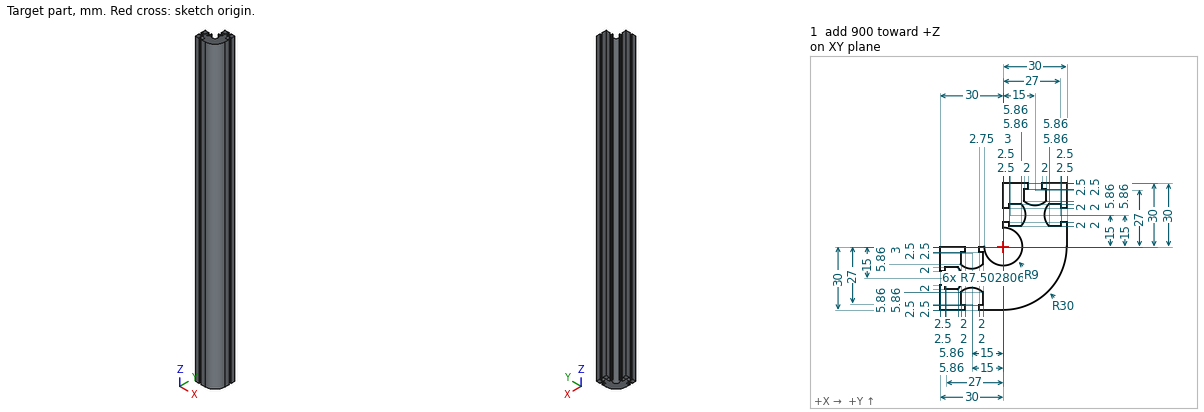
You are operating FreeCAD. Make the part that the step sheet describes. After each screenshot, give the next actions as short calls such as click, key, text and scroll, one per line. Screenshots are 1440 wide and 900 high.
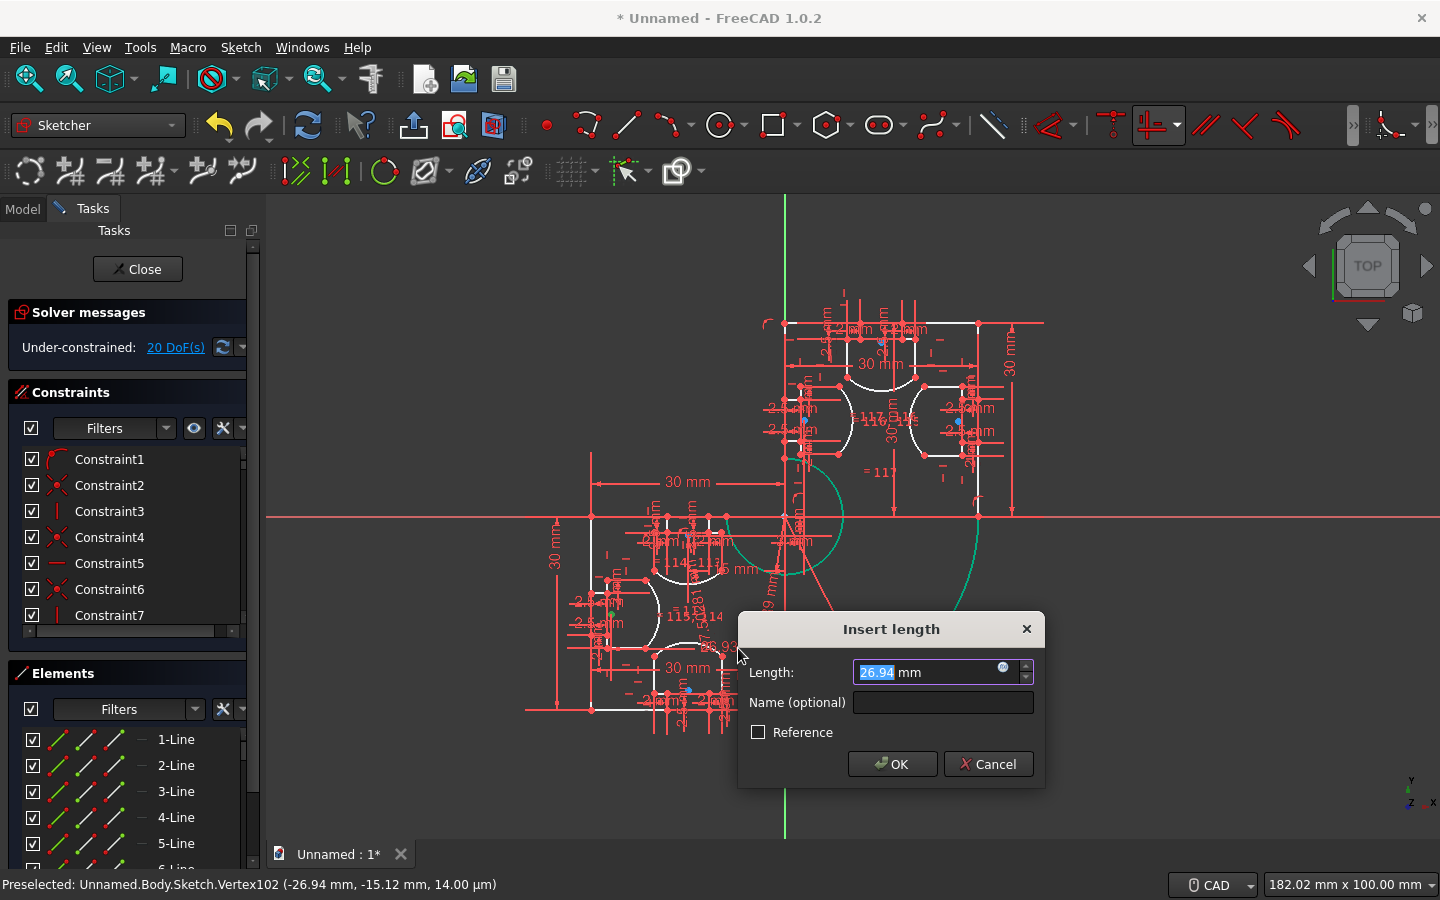
text(27)
key(Return)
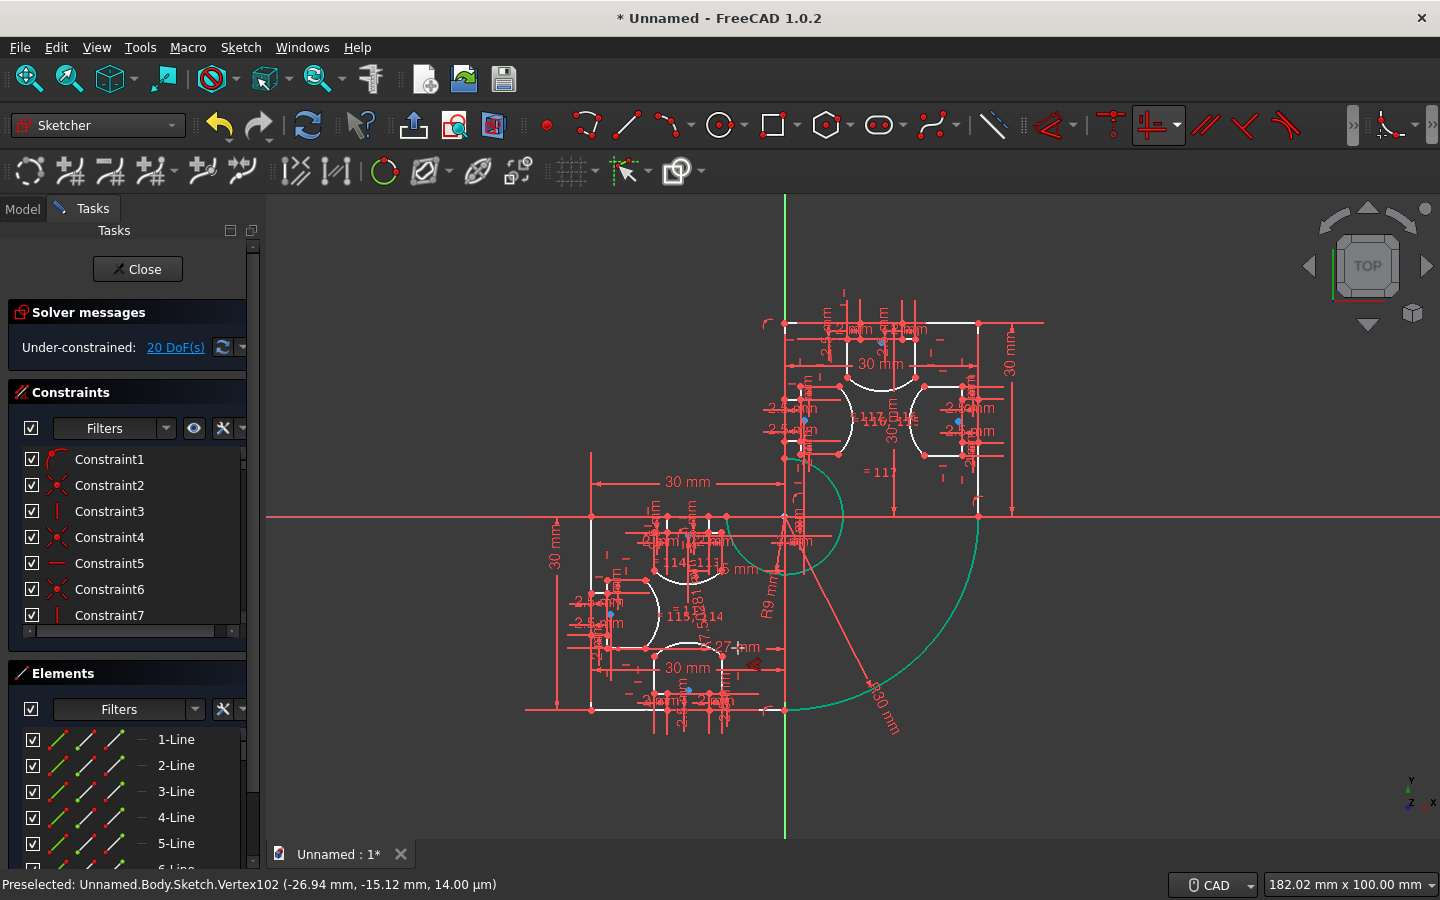
click(611, 614)
click(843, 565)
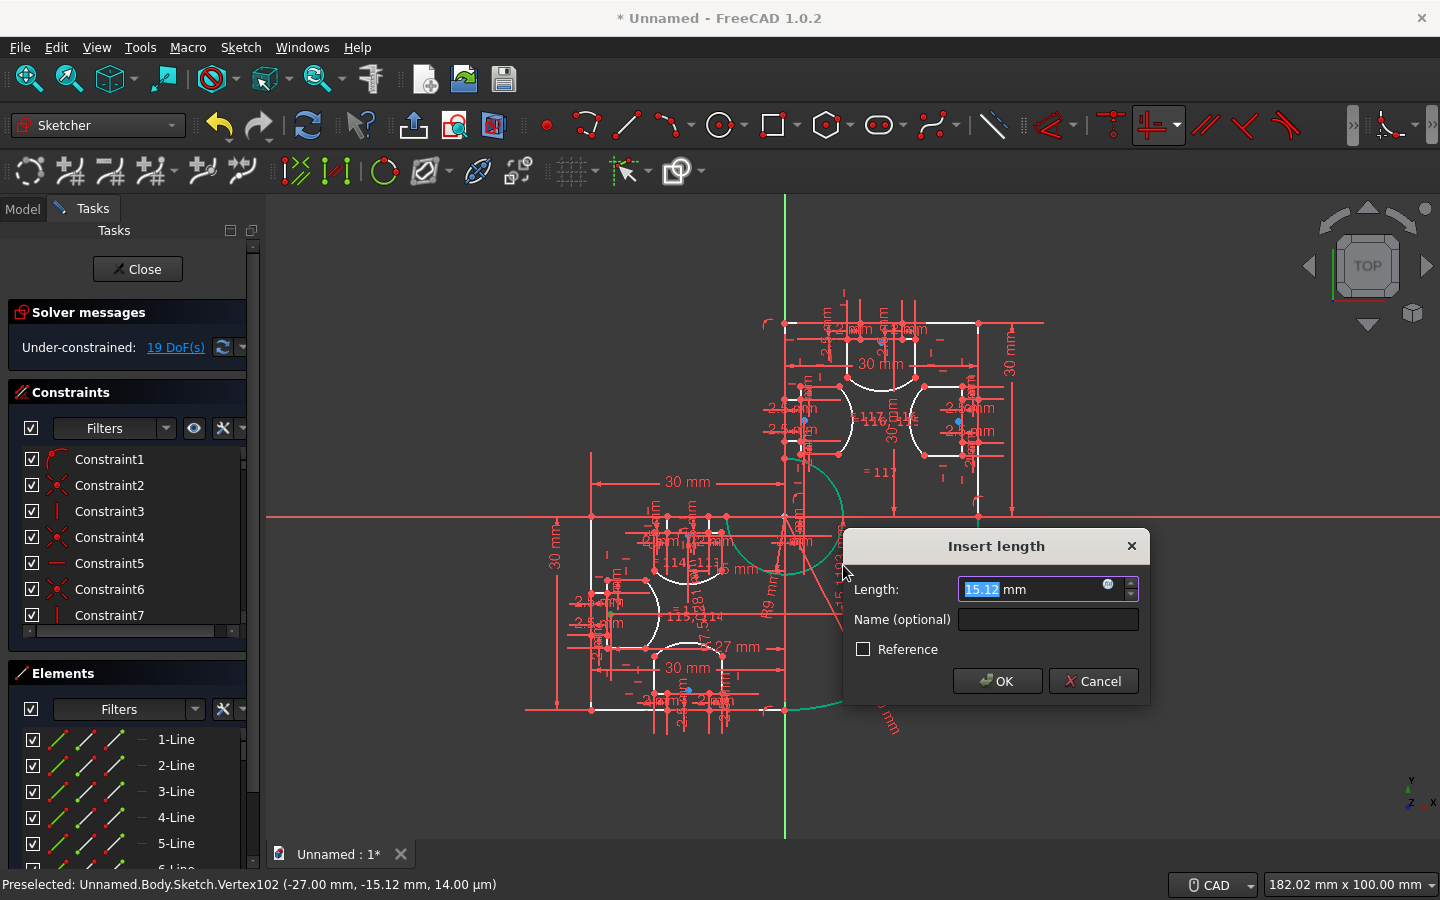
text(15)
key(Return)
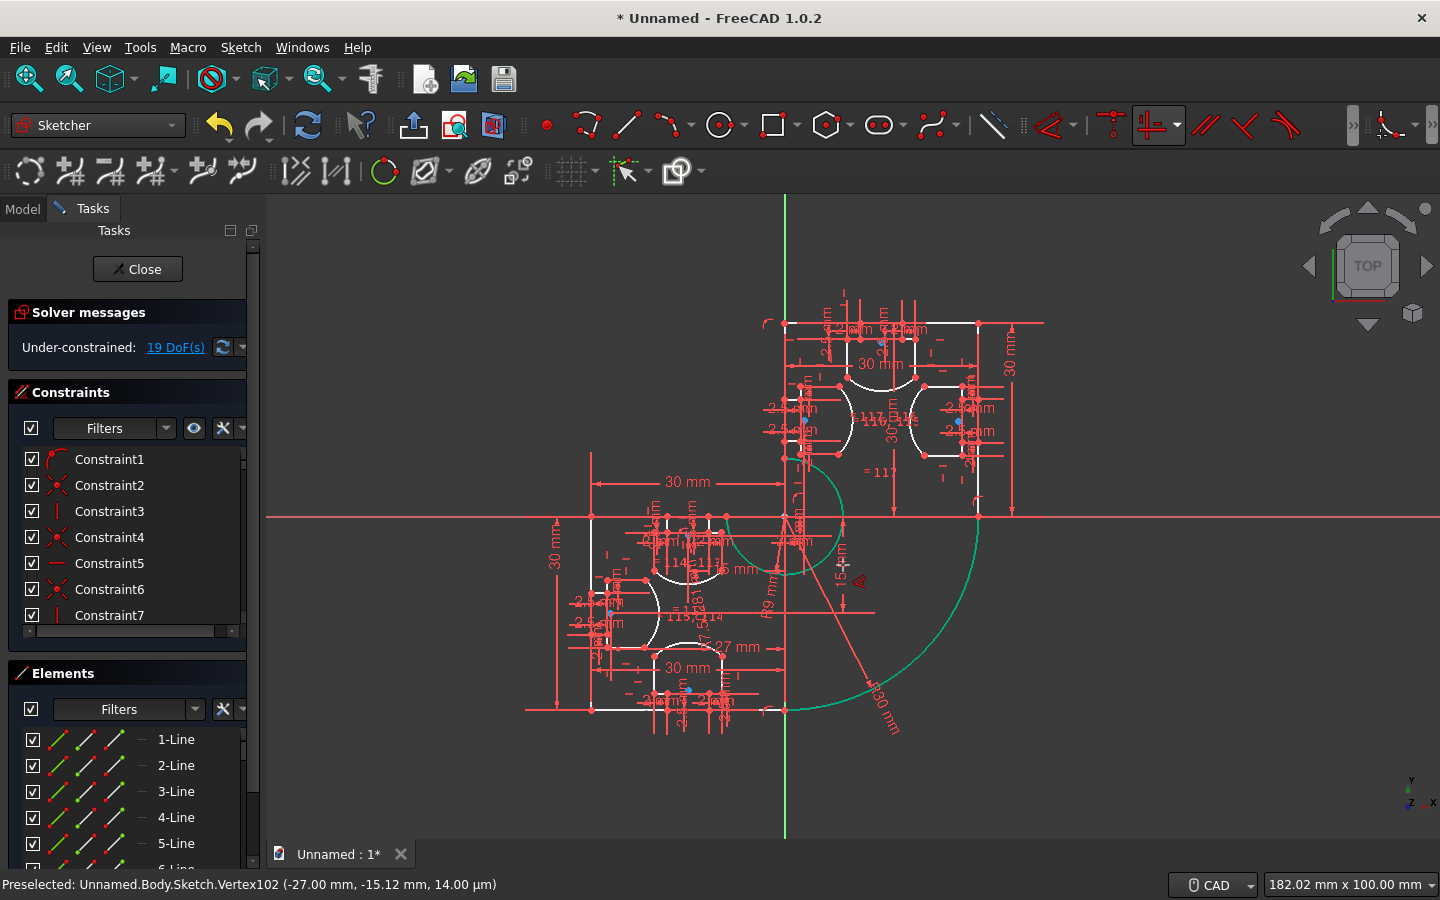
click(688, 691)
click(737, 725)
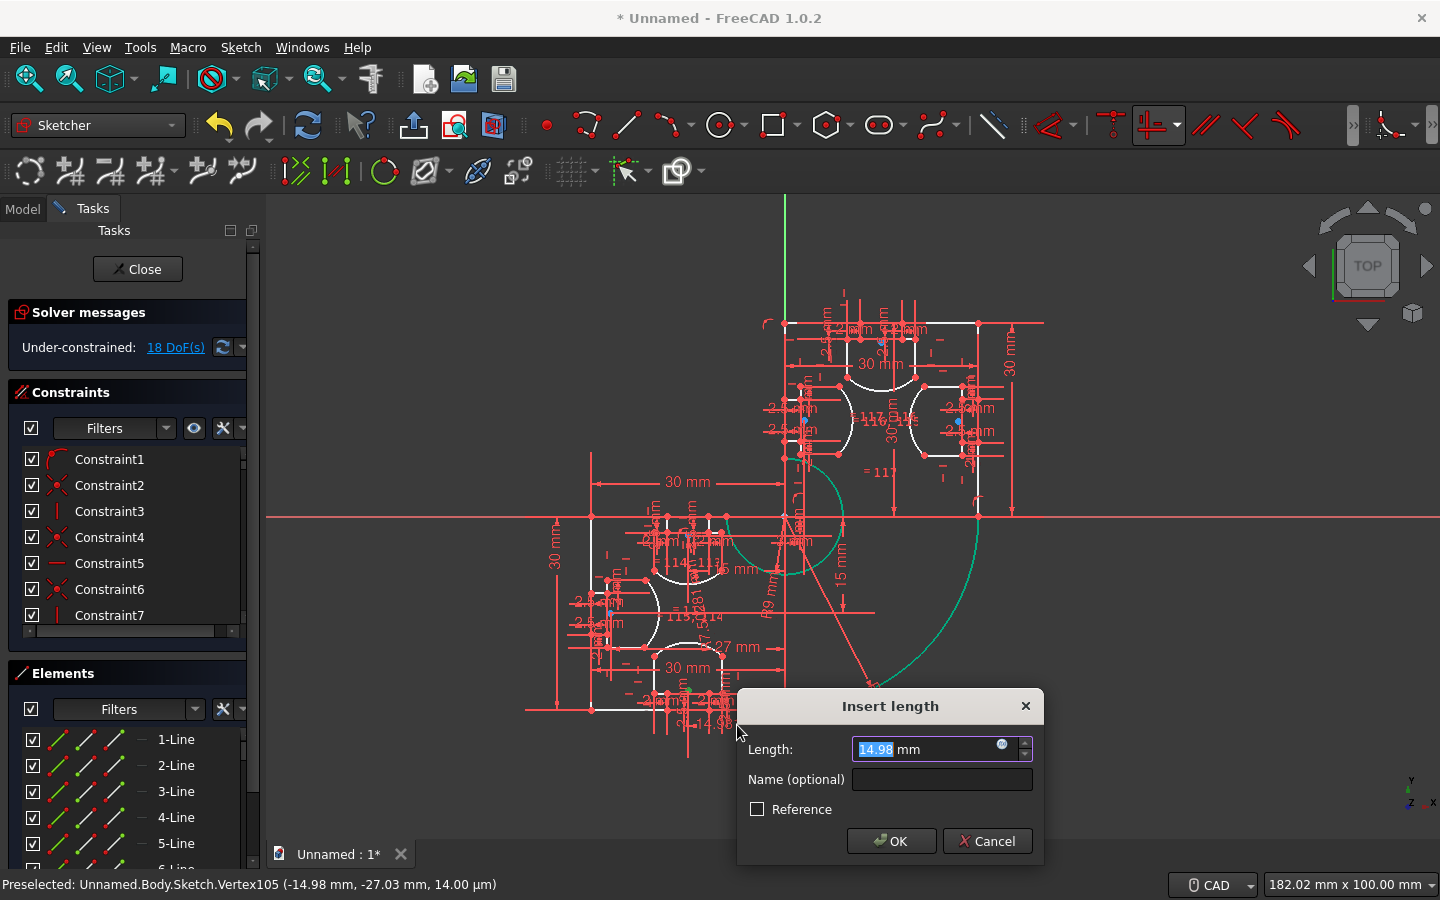
text(15)
key(Return)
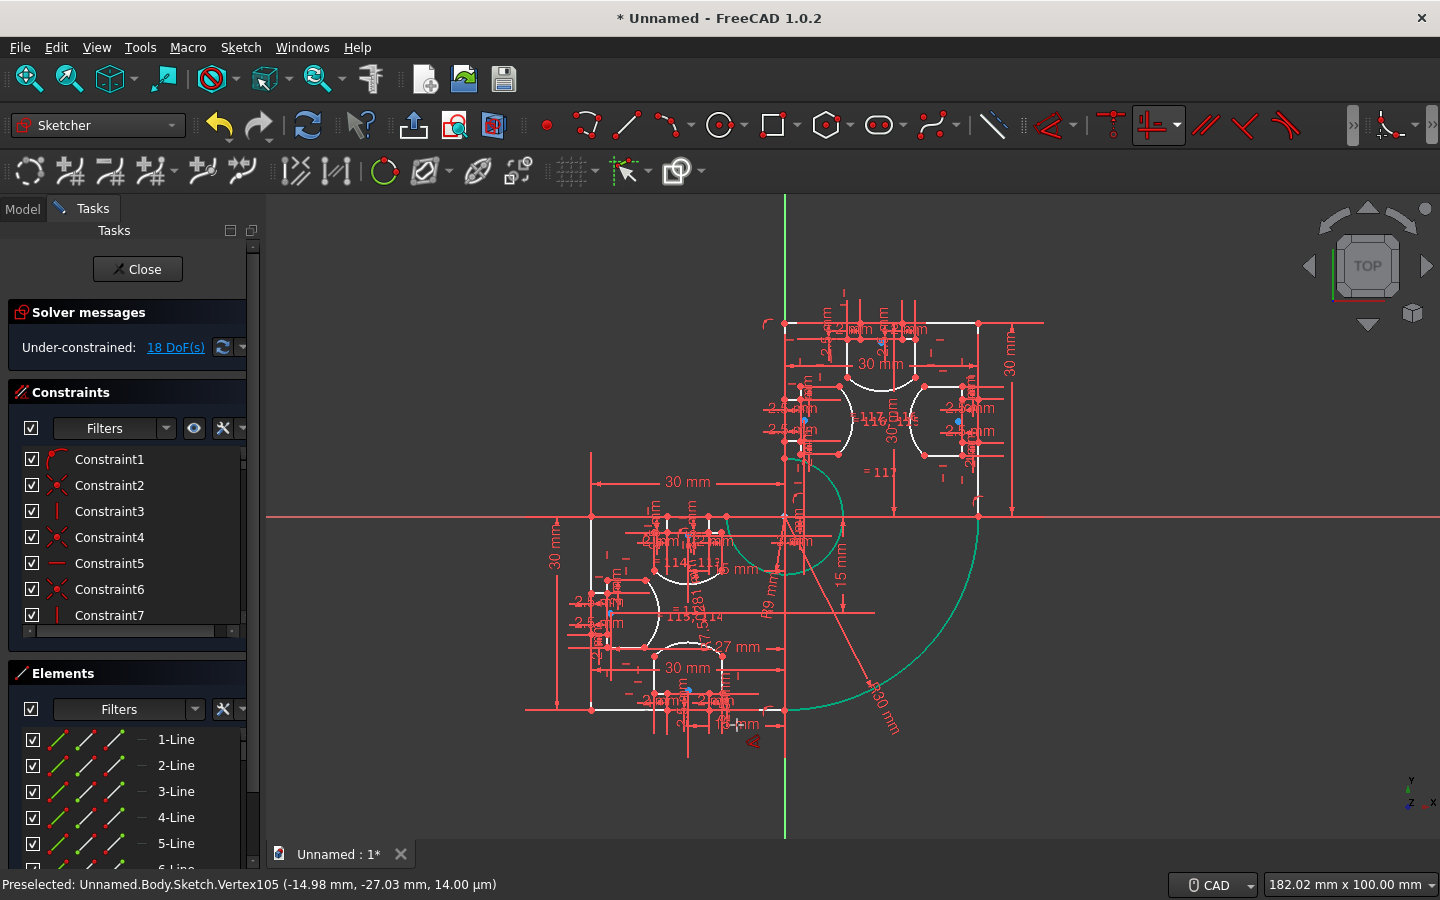
click(688, 691)
click(819, 644)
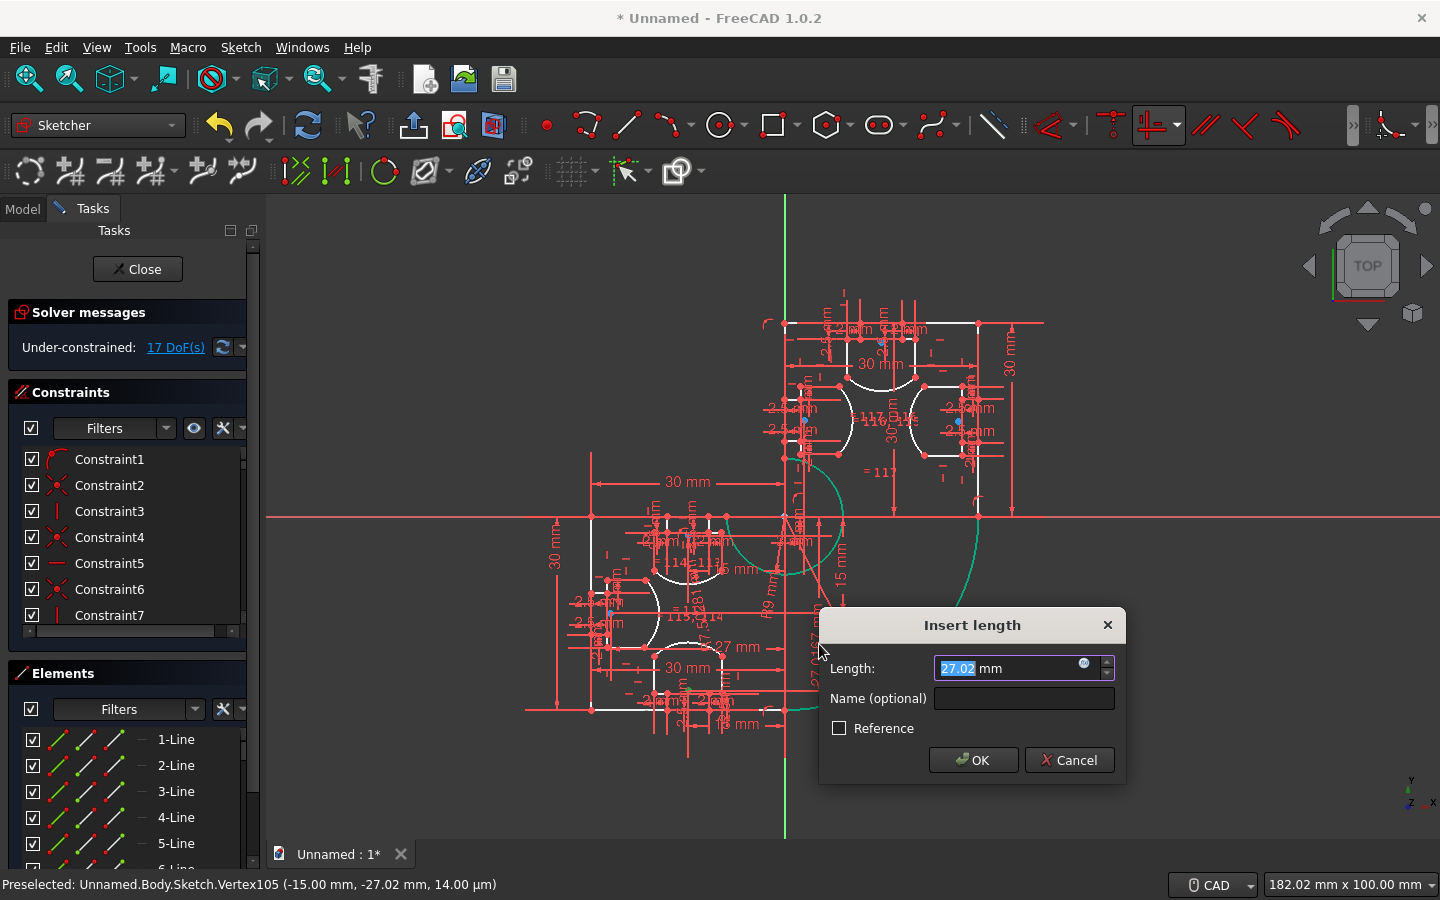
text(27)
key(Return)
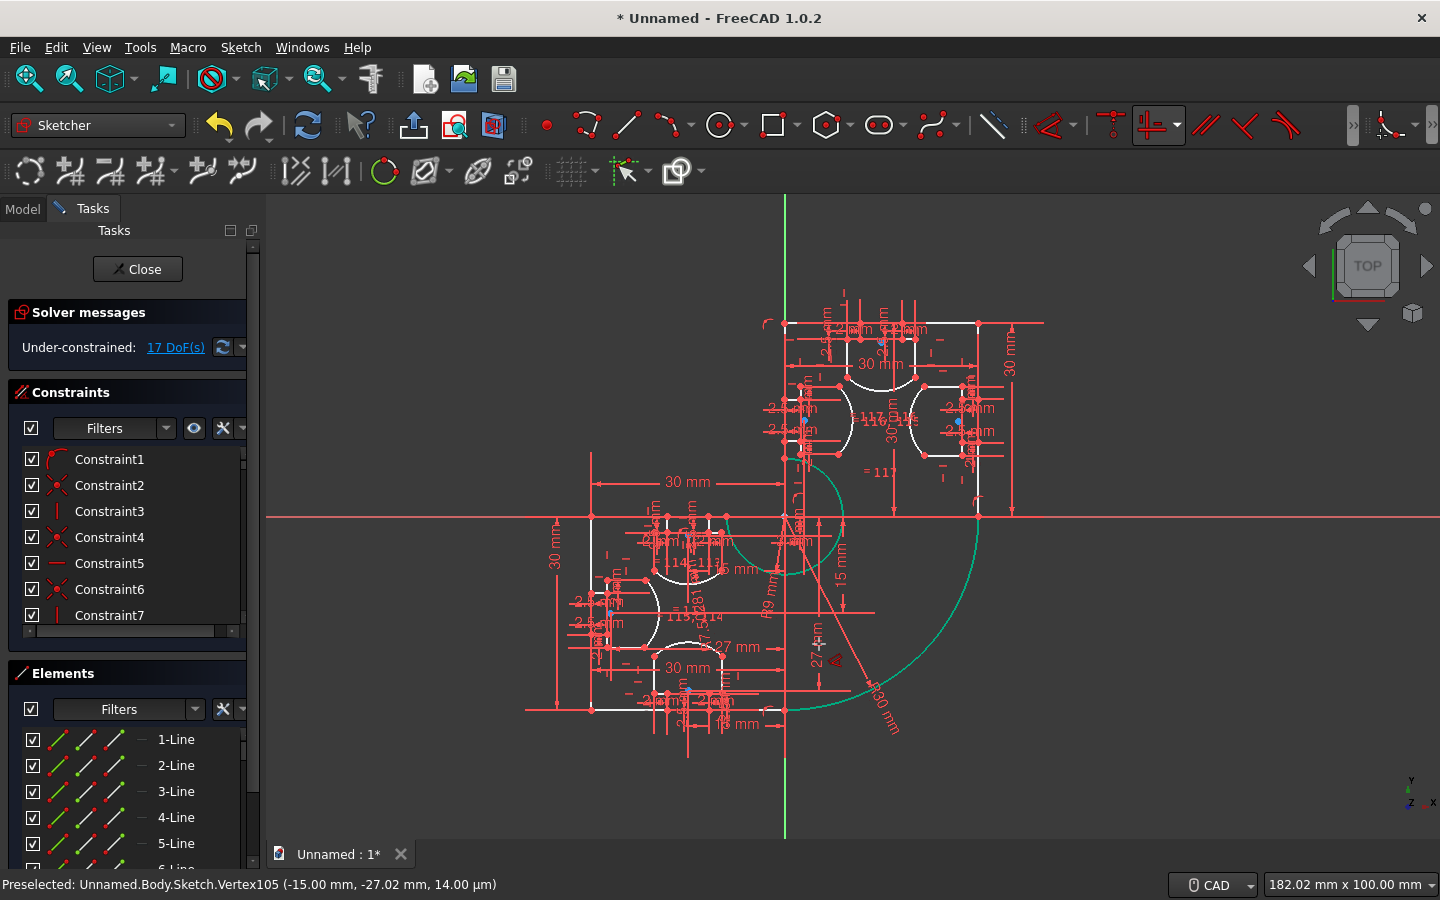
click(958, 421)
click(932, 551)